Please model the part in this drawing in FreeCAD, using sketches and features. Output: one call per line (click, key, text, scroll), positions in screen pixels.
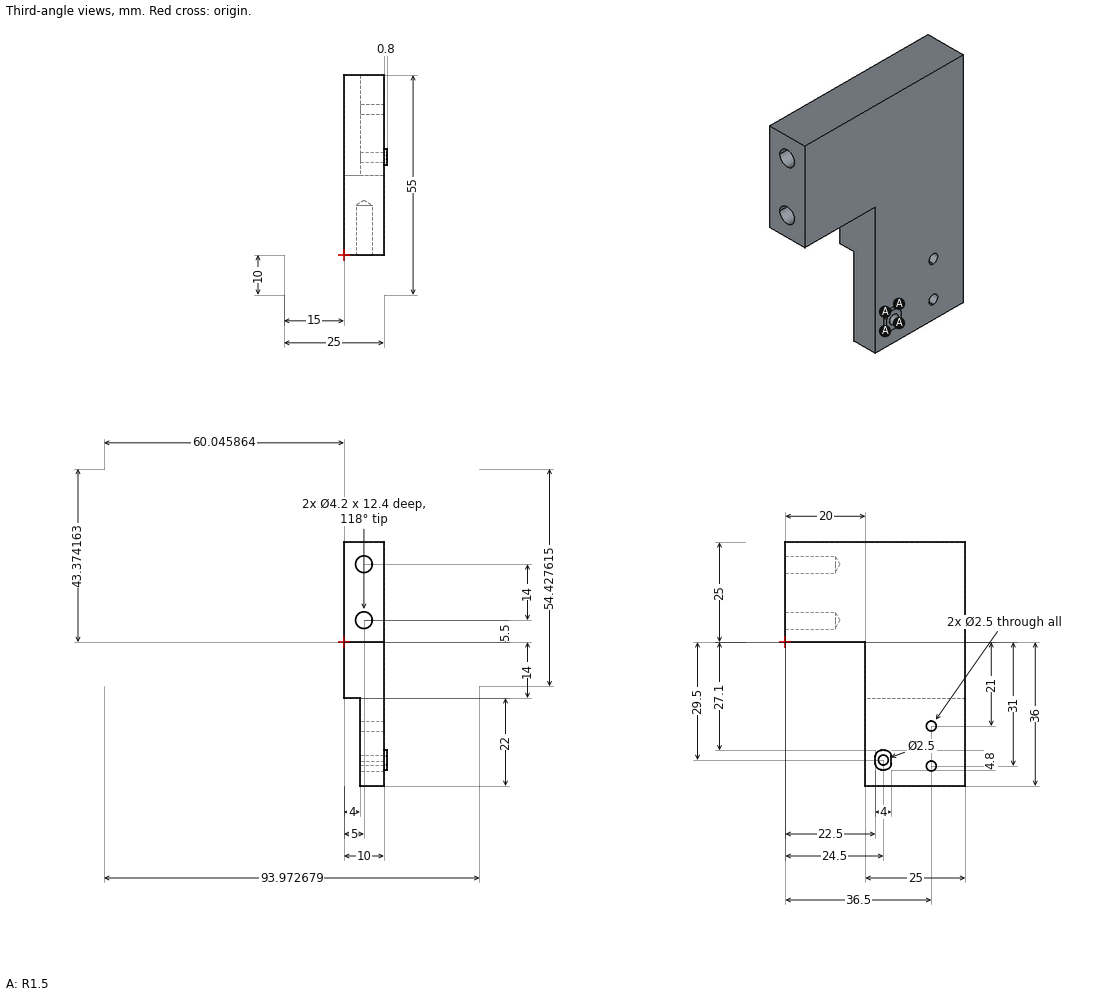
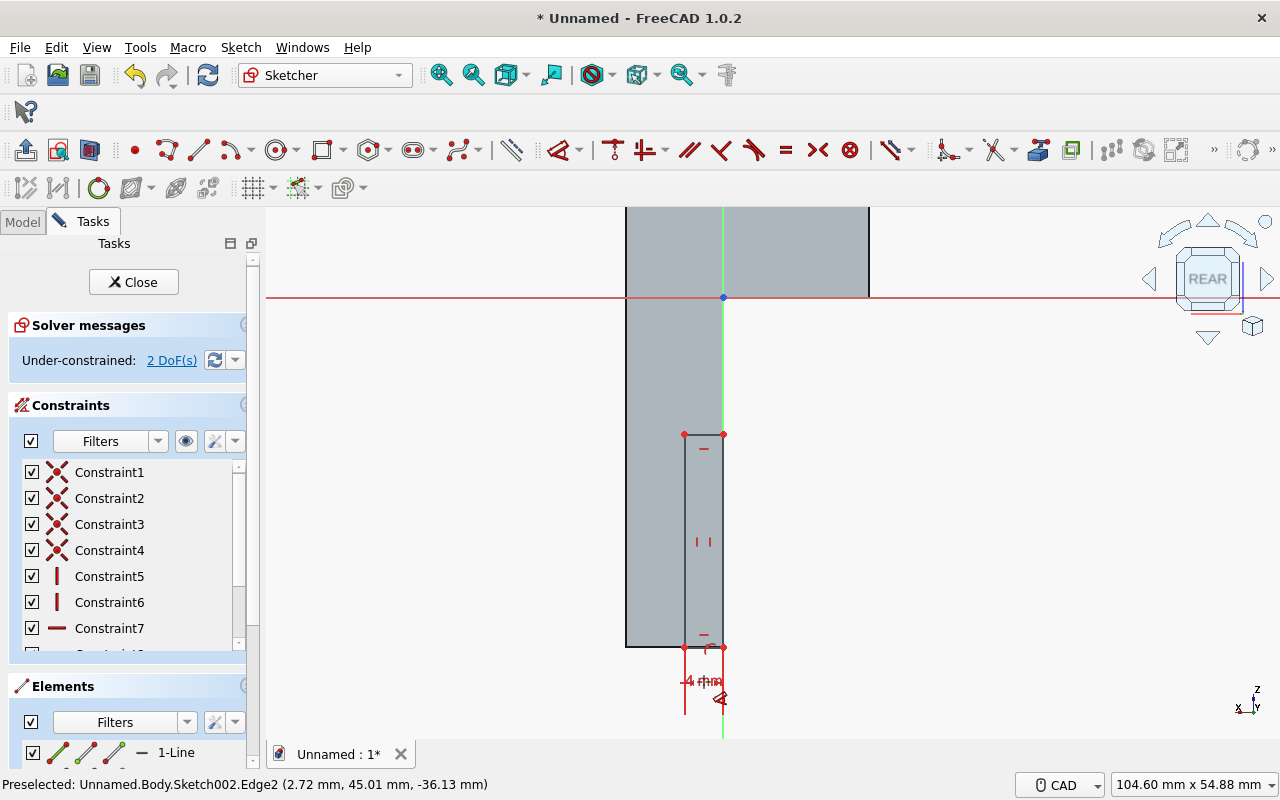
click(685, 499)
click(651, 541)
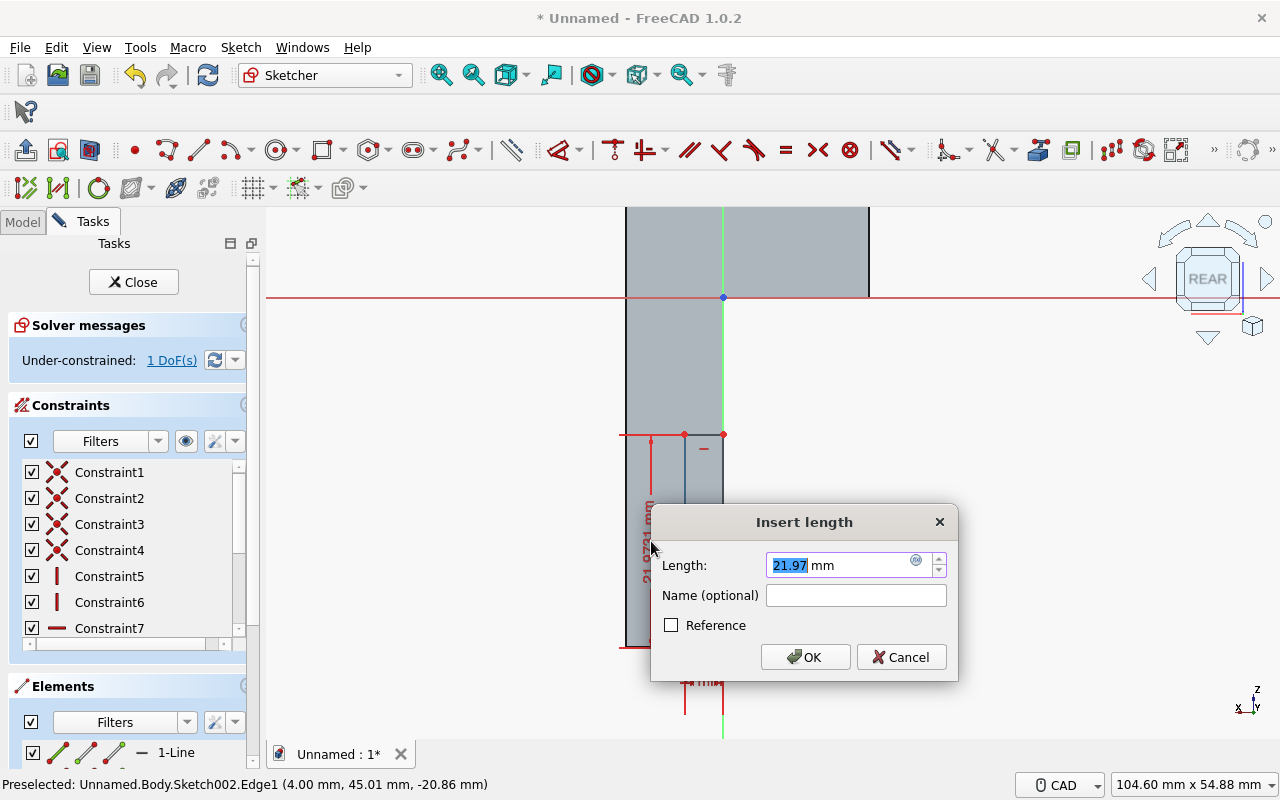
text(22)
key(Return)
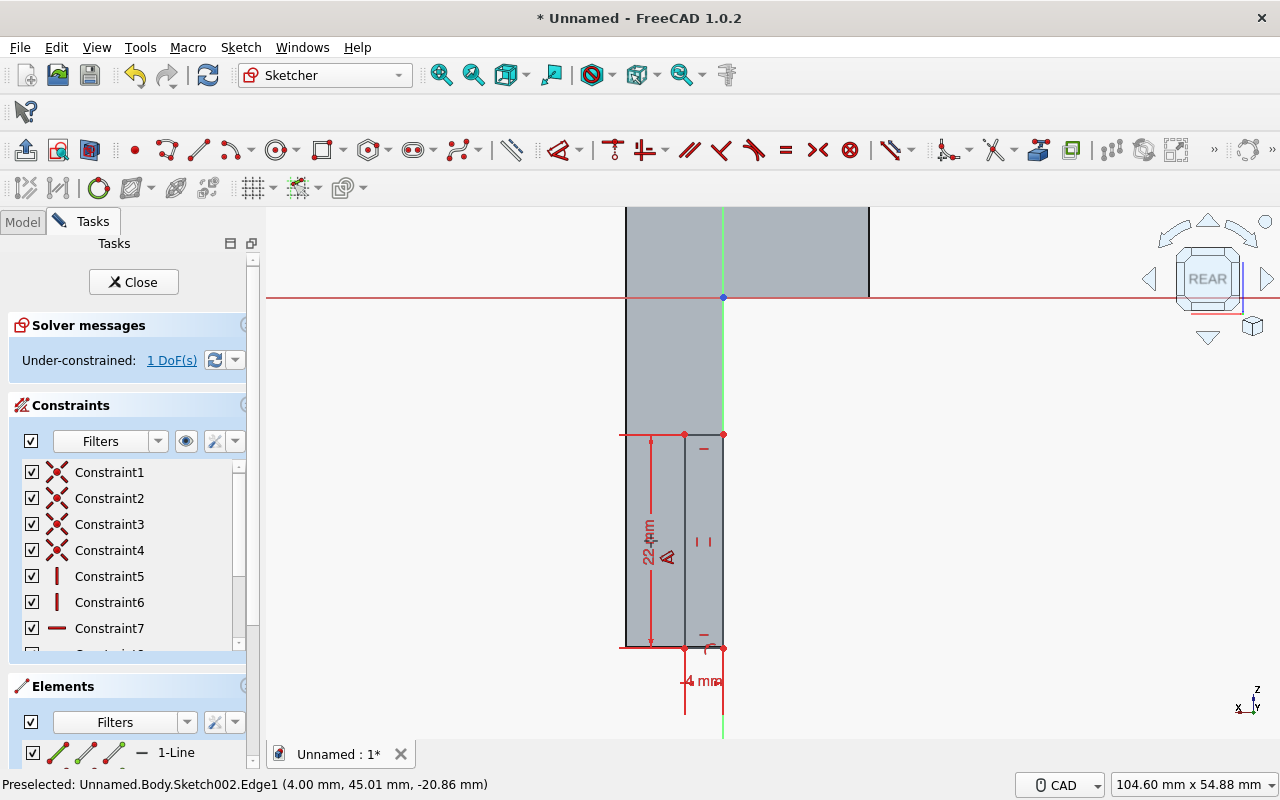
click(685, 435)
click(651, 366)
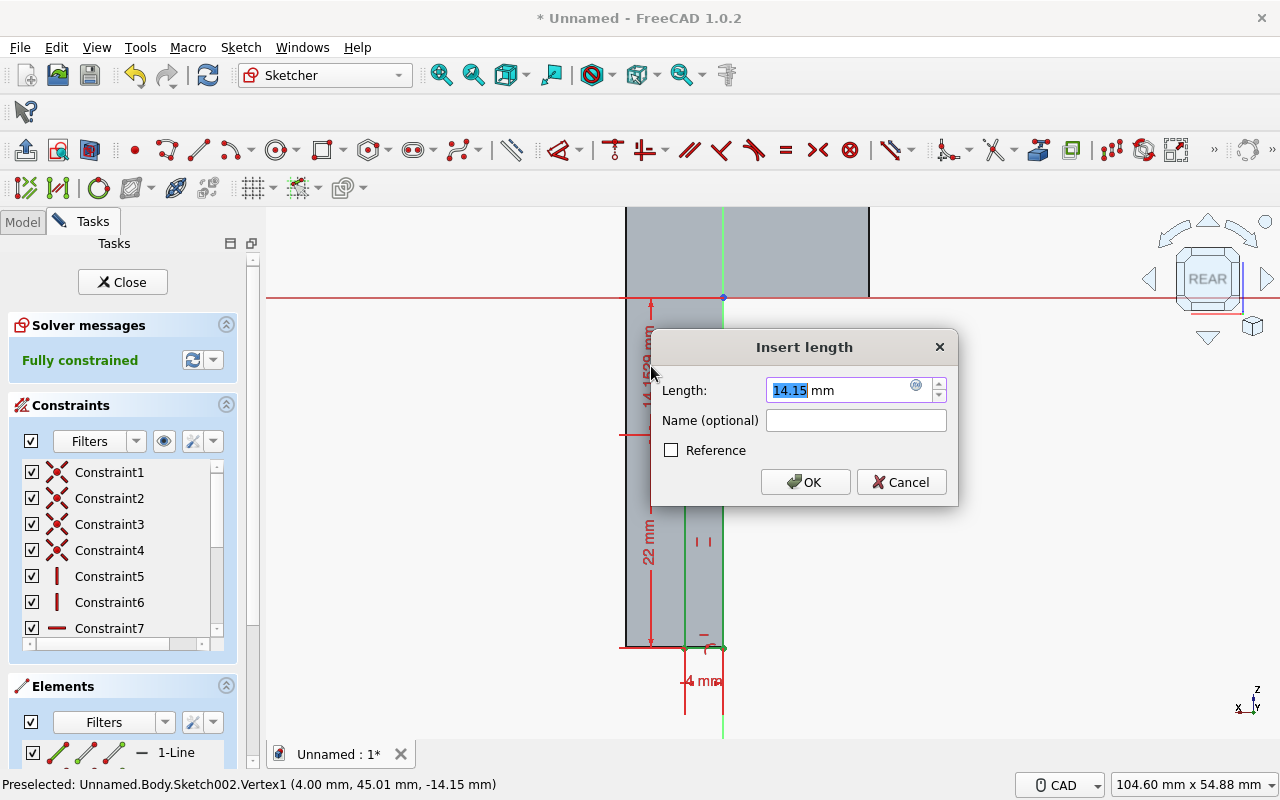
text(14)
key(Return)
key(Escape)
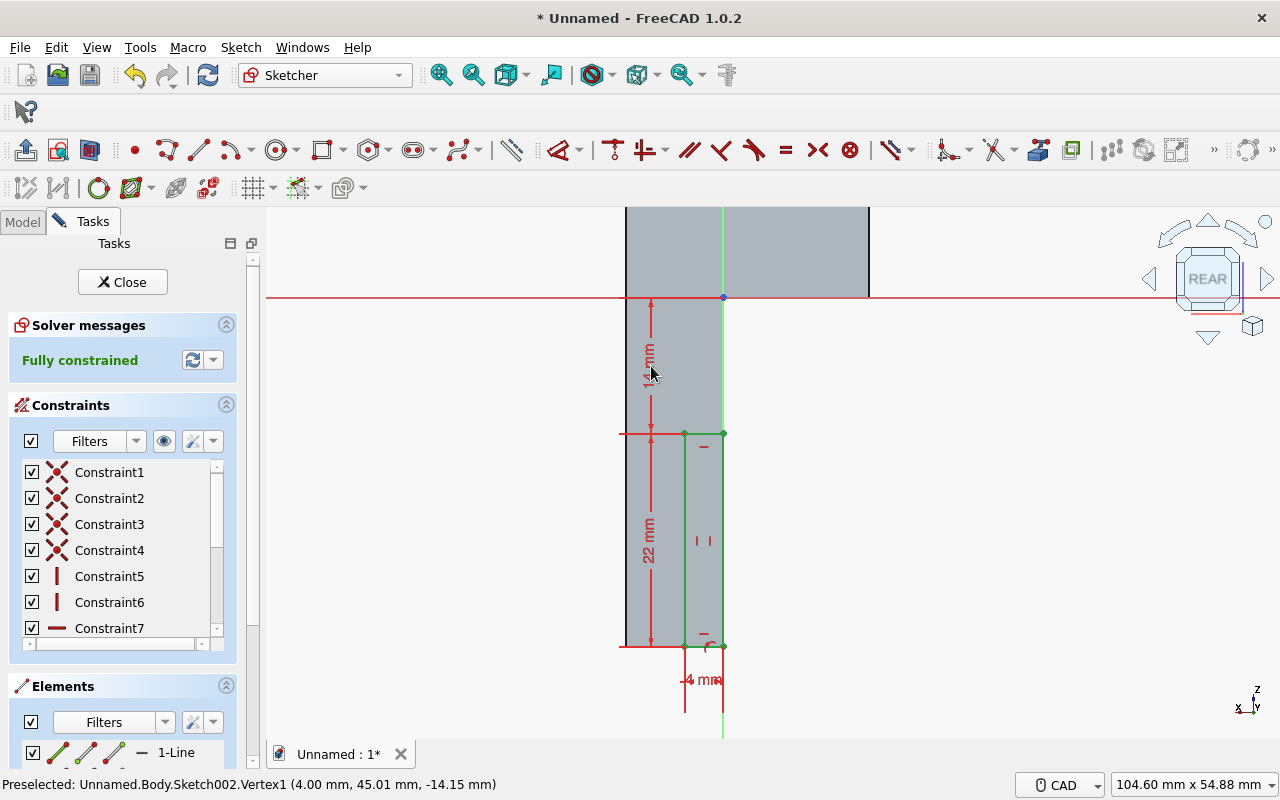
click(123, 282)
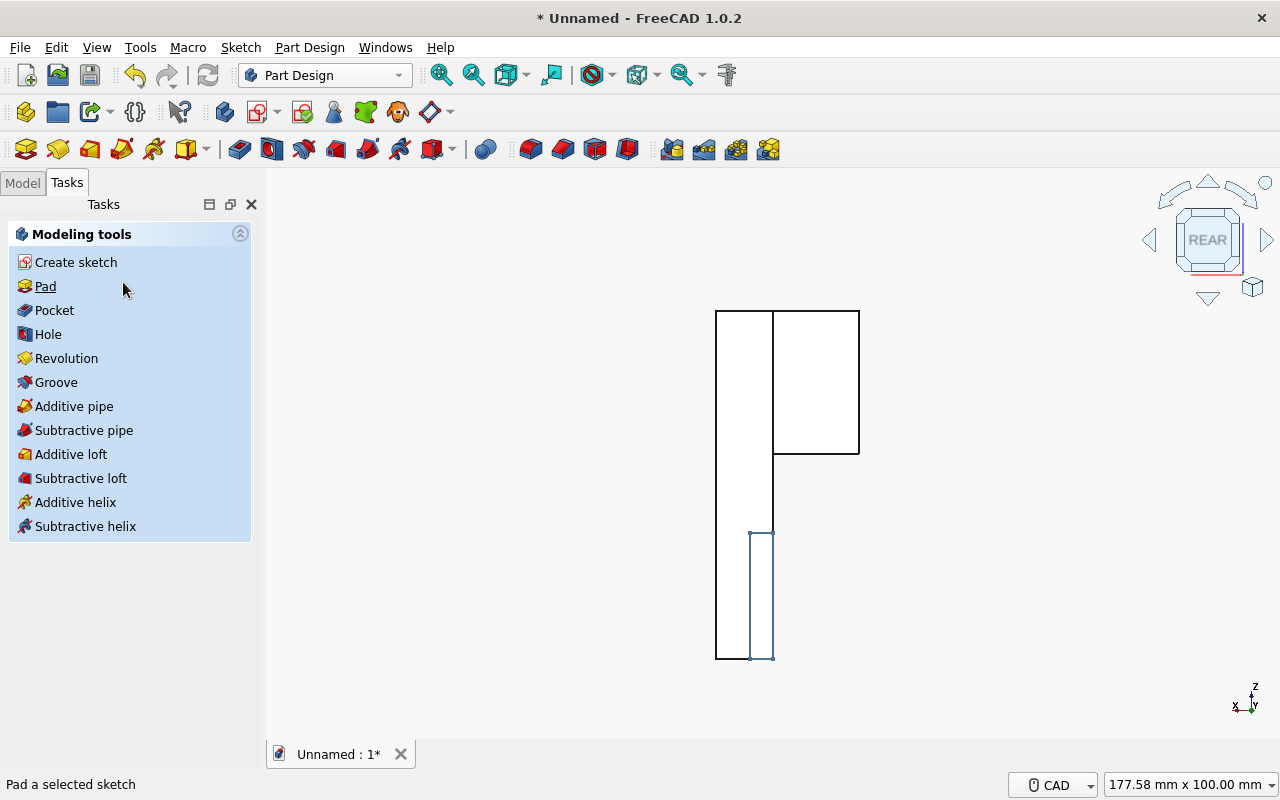
click(240, 150)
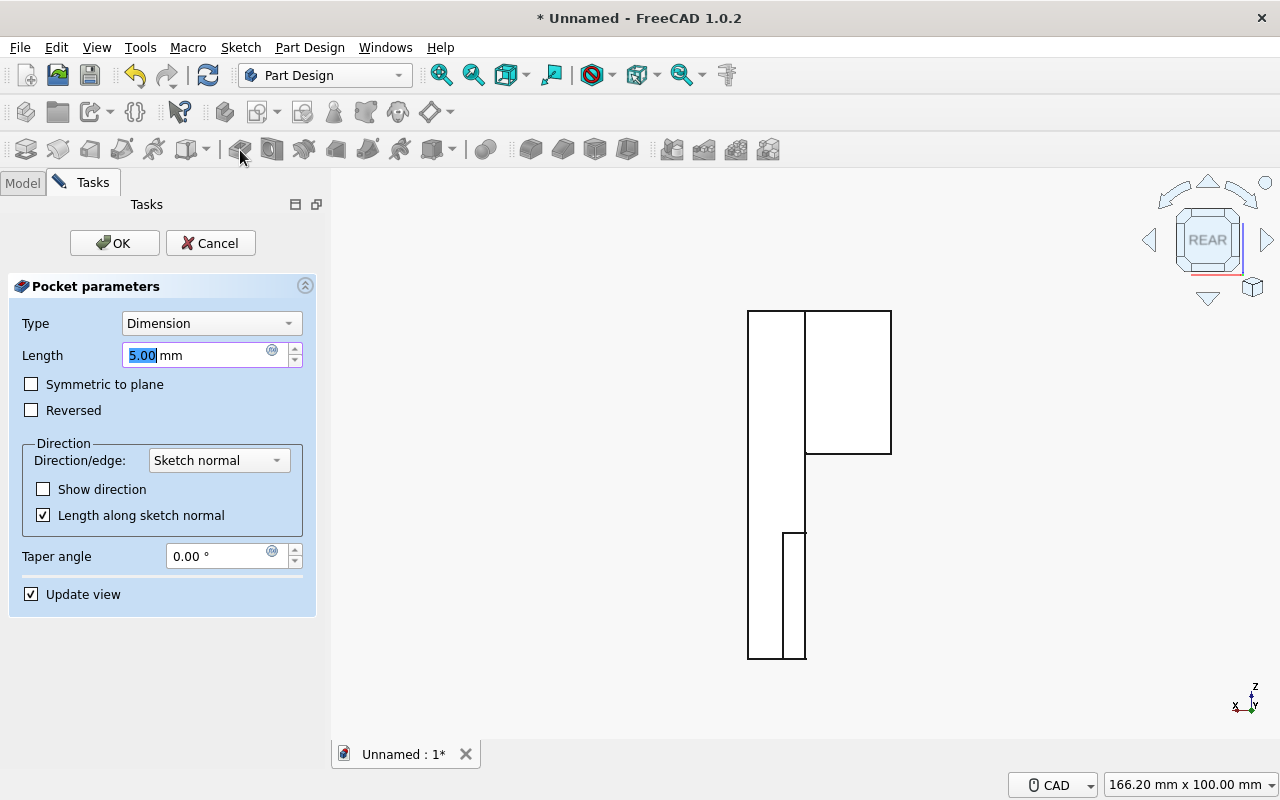
click(212, 324)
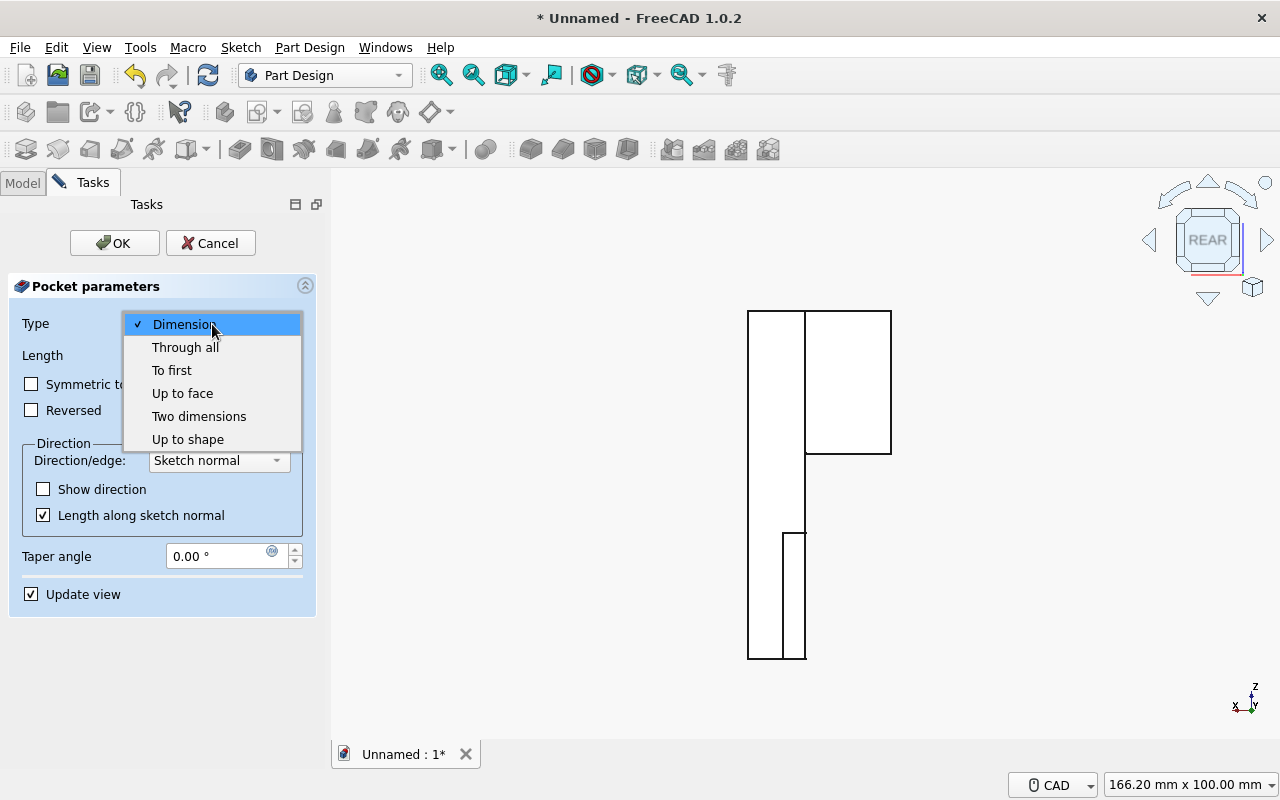
click(212, 348)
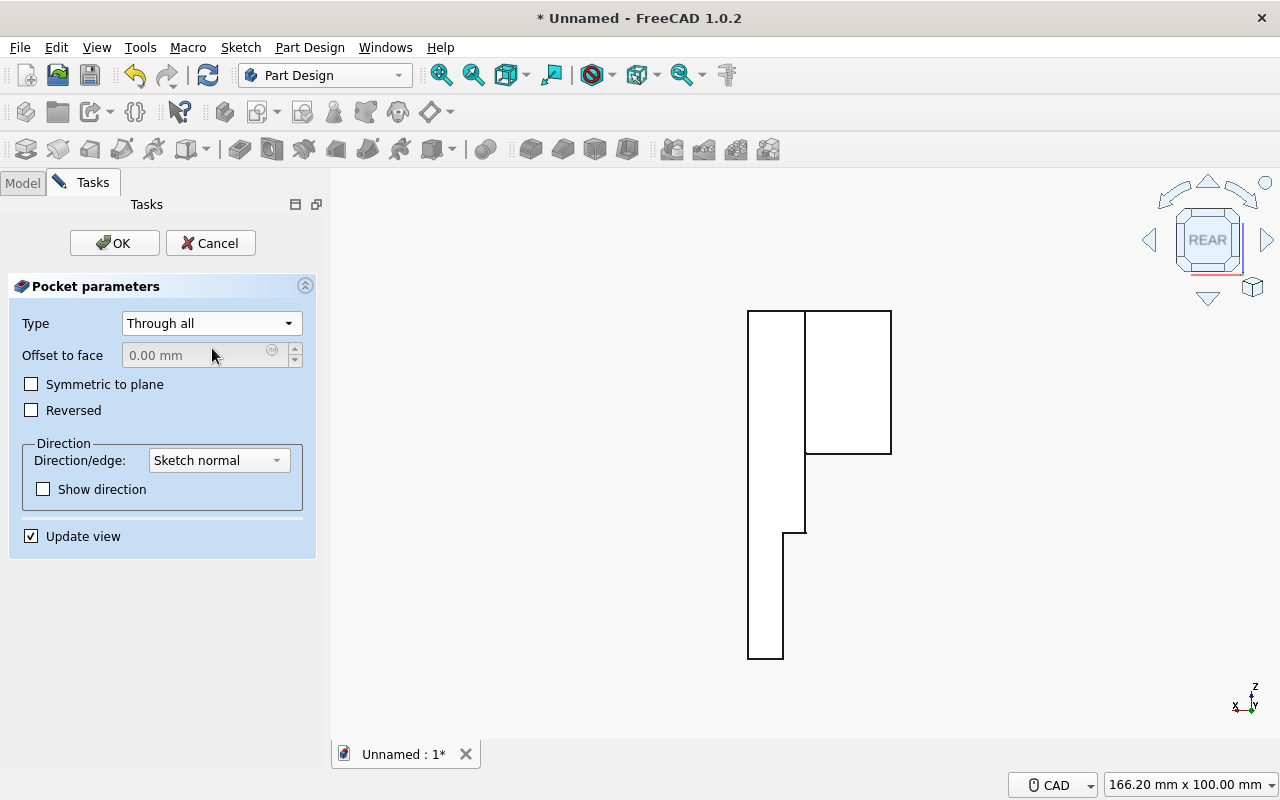
click(115, 243)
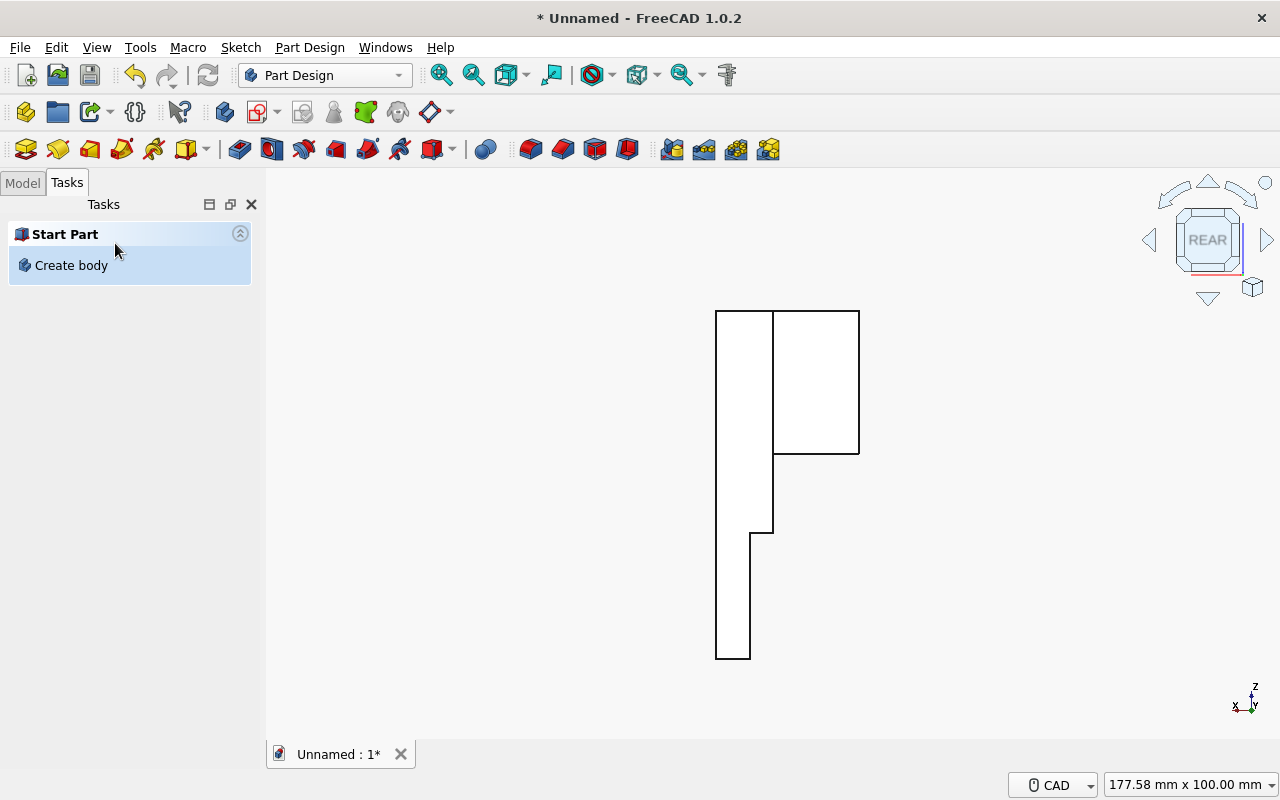
key(0)